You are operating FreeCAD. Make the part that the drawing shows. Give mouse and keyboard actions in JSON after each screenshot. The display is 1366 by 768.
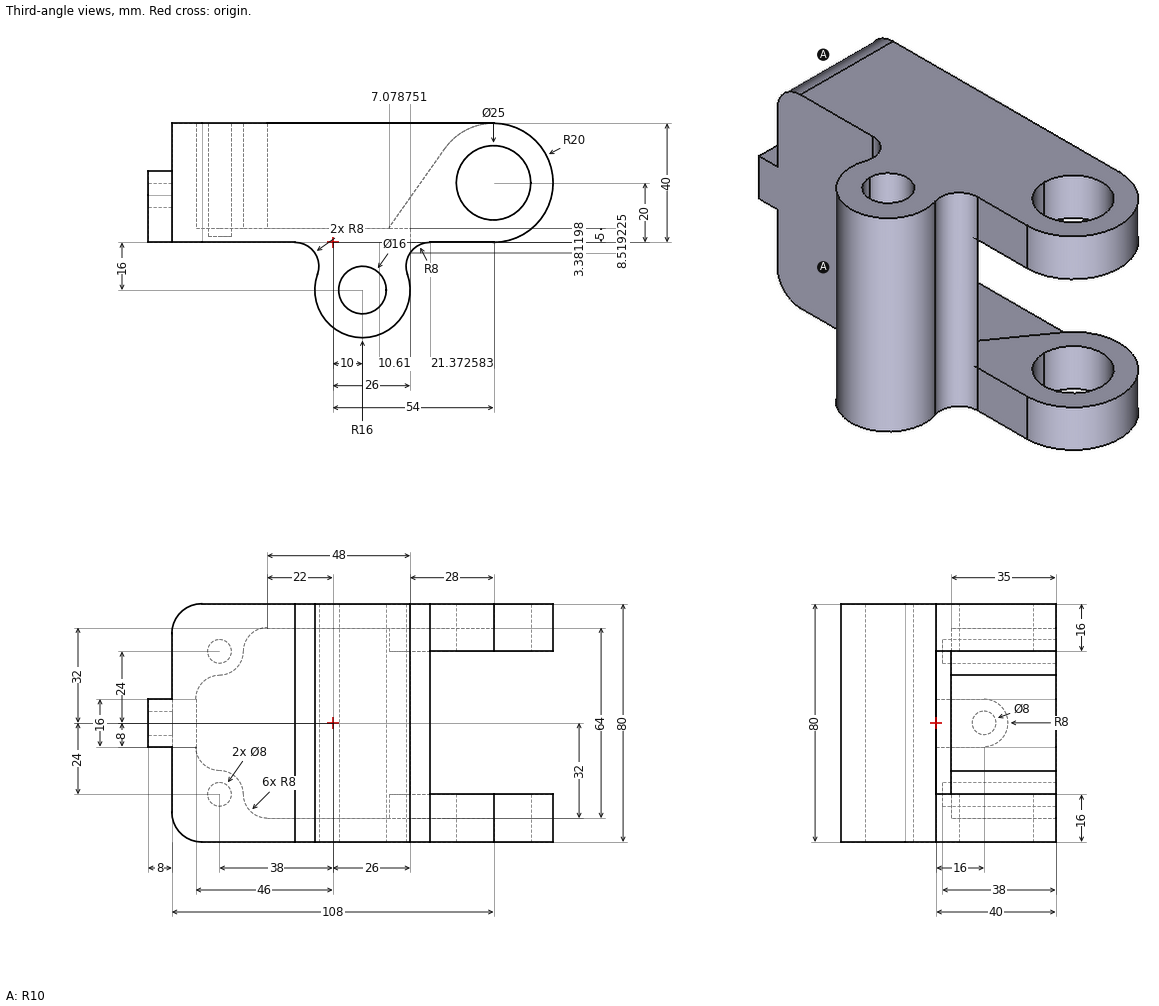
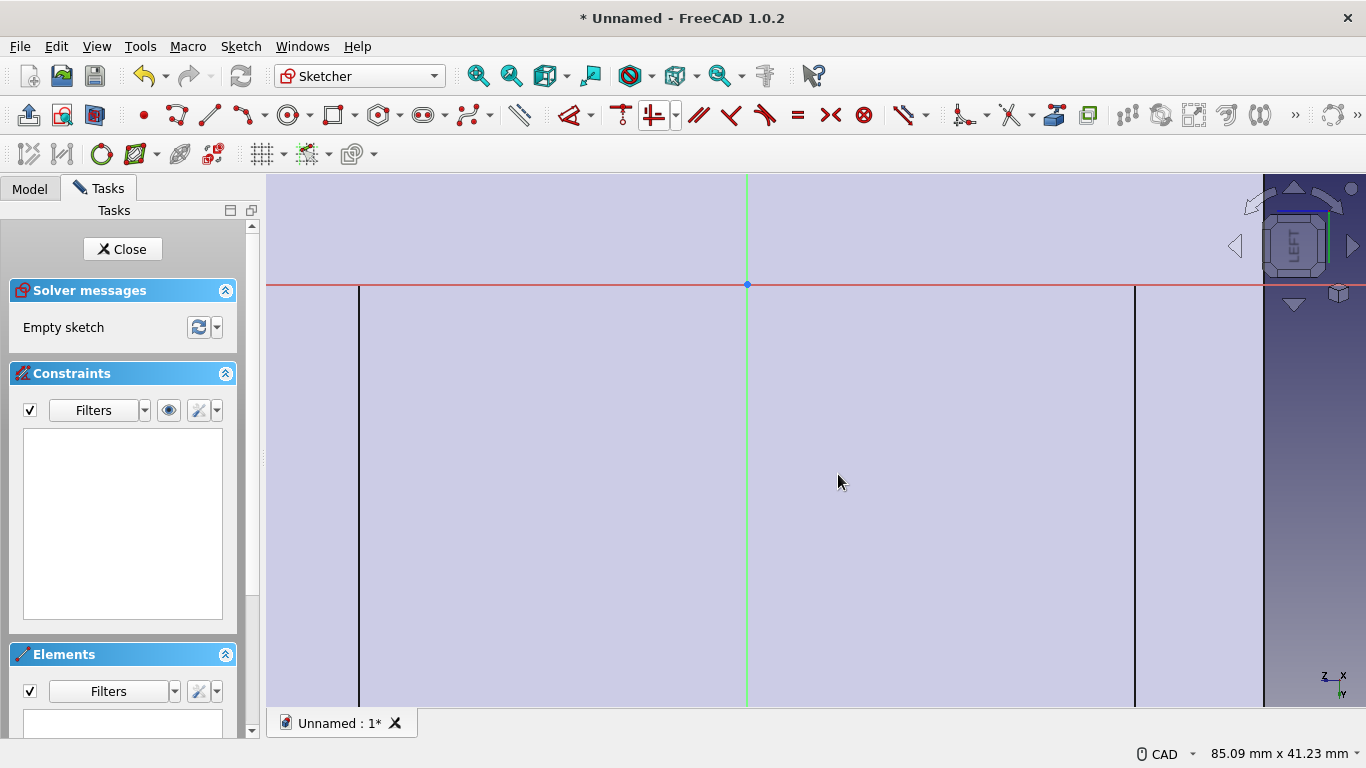
{"action": "key", "text": "g m"}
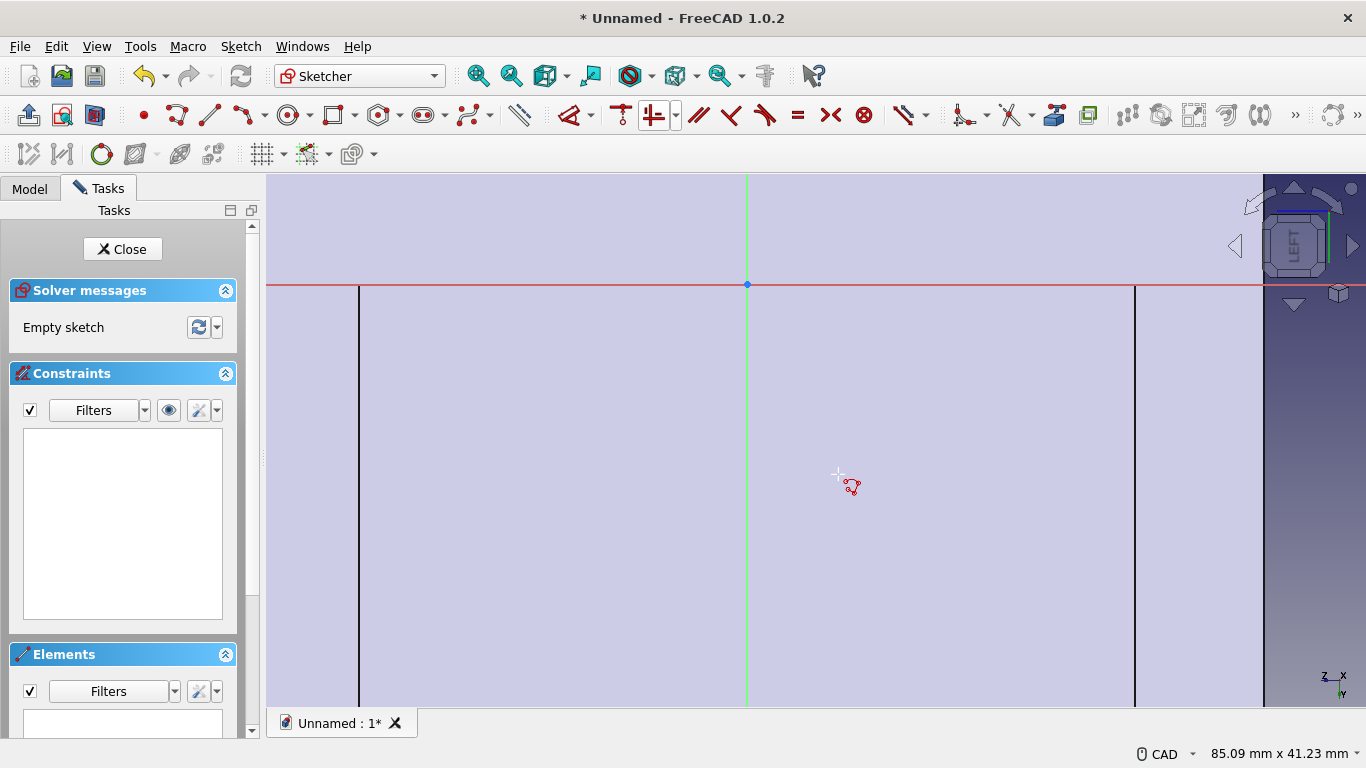
{"action": "left_click", "coordinate": [851, 492]}
{"action": "left_click", "coordinate": [851, 285]}
{"action": "left_click", "coordinate": [644, 294]}
{"action": "left_click", "coordinate": [644, 492]}
{"action": "right_click", "coordinate": [644, 492]}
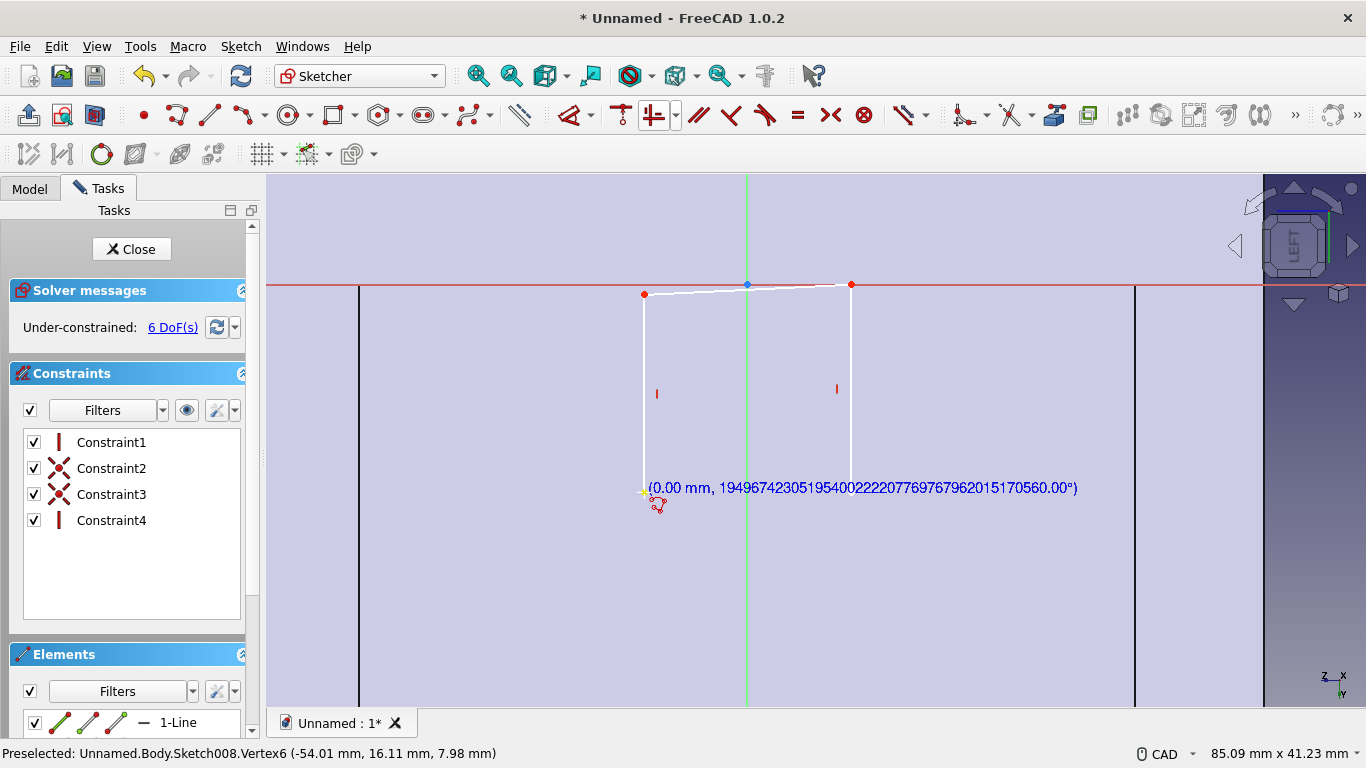
{"action": "left_click", "coordinate": [242, 116]}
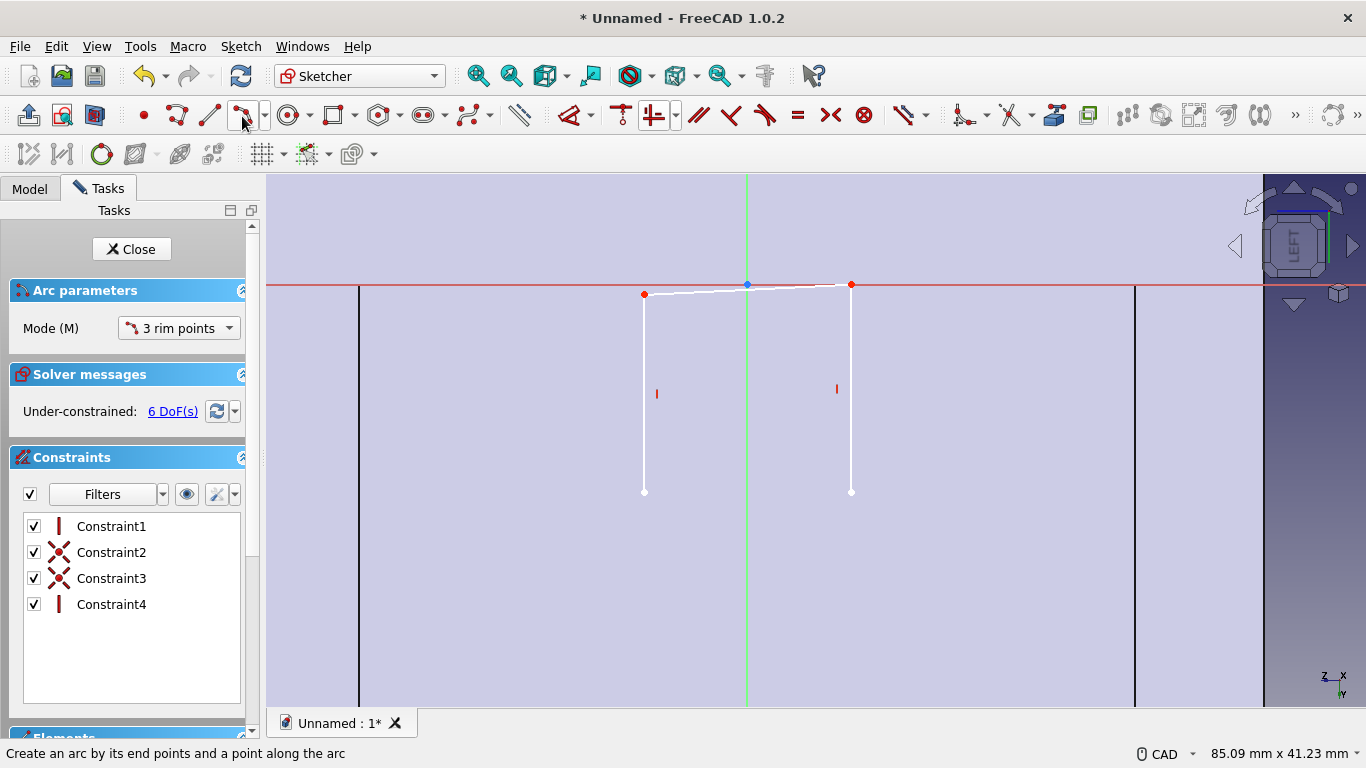
{"action": "left_click", "coordinate": [644, 493]}
{"action": "left_click", "coordinate": [851, 493]}
{"action": "left_click", "coordinate": [715, 590]}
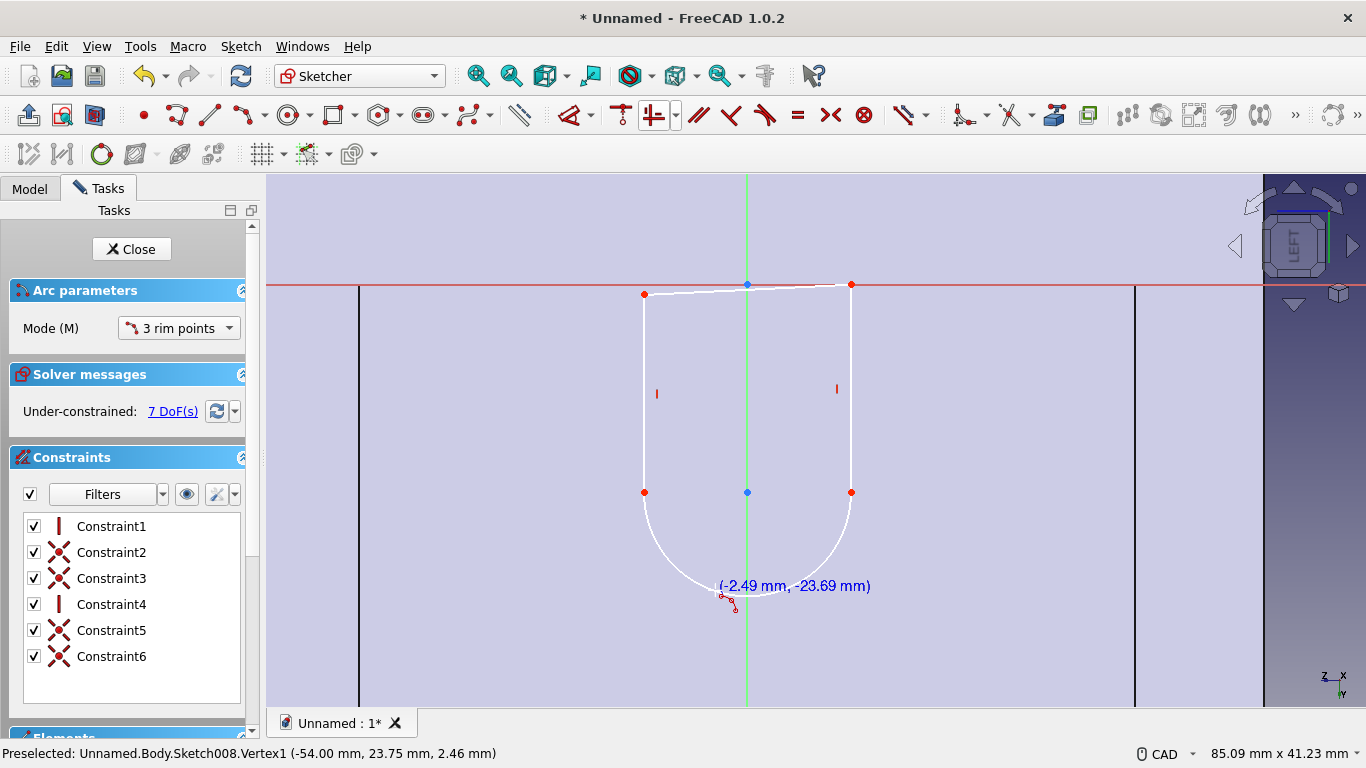
{"action": "key", "text": "g c"}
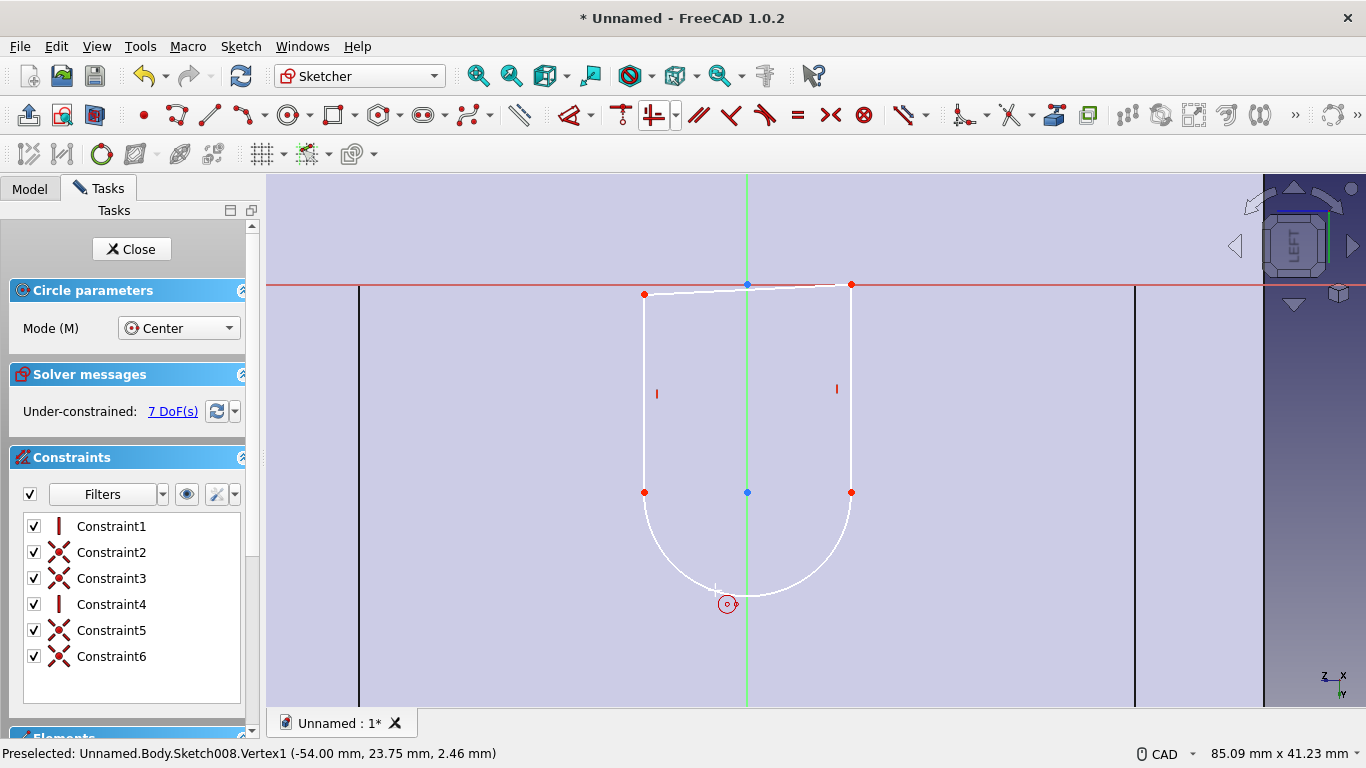
{"action": "left_click", "coordinate": [747, 492]}
{"action": "mouse_move", "coordinate": [784, 455]}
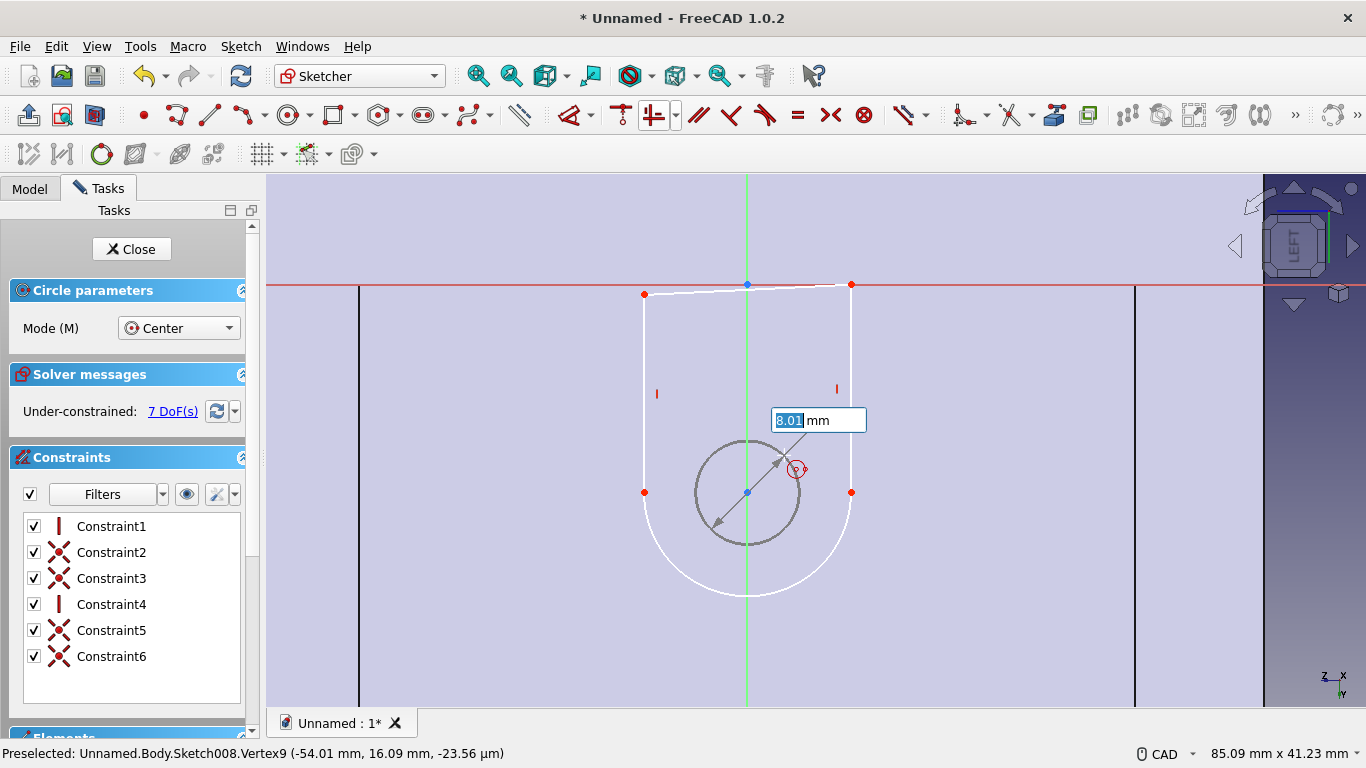
{"action": "type", "text": "8"}
{"action": "key", "text": "Return"}
{"action": "key", "text": "Escape"}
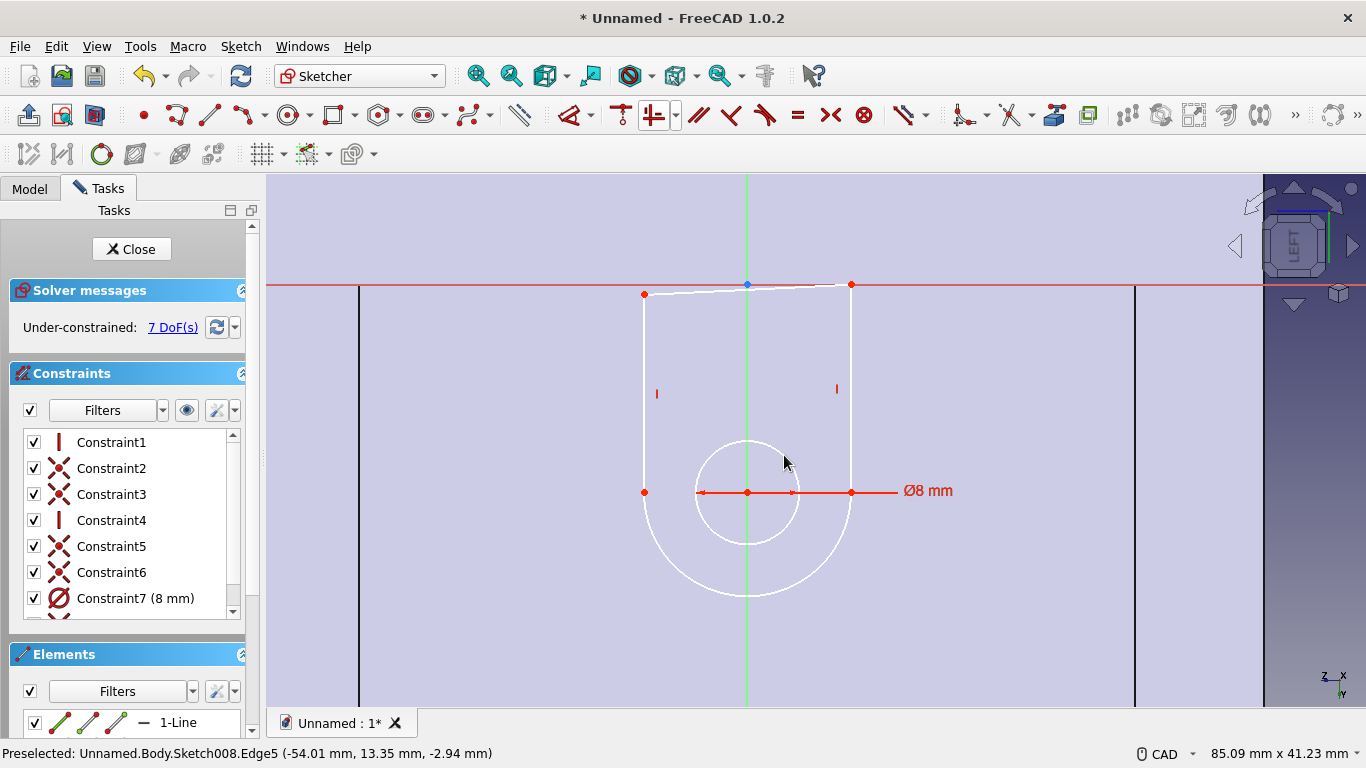
{"action": "left_click", "coordinate": [851, 431]}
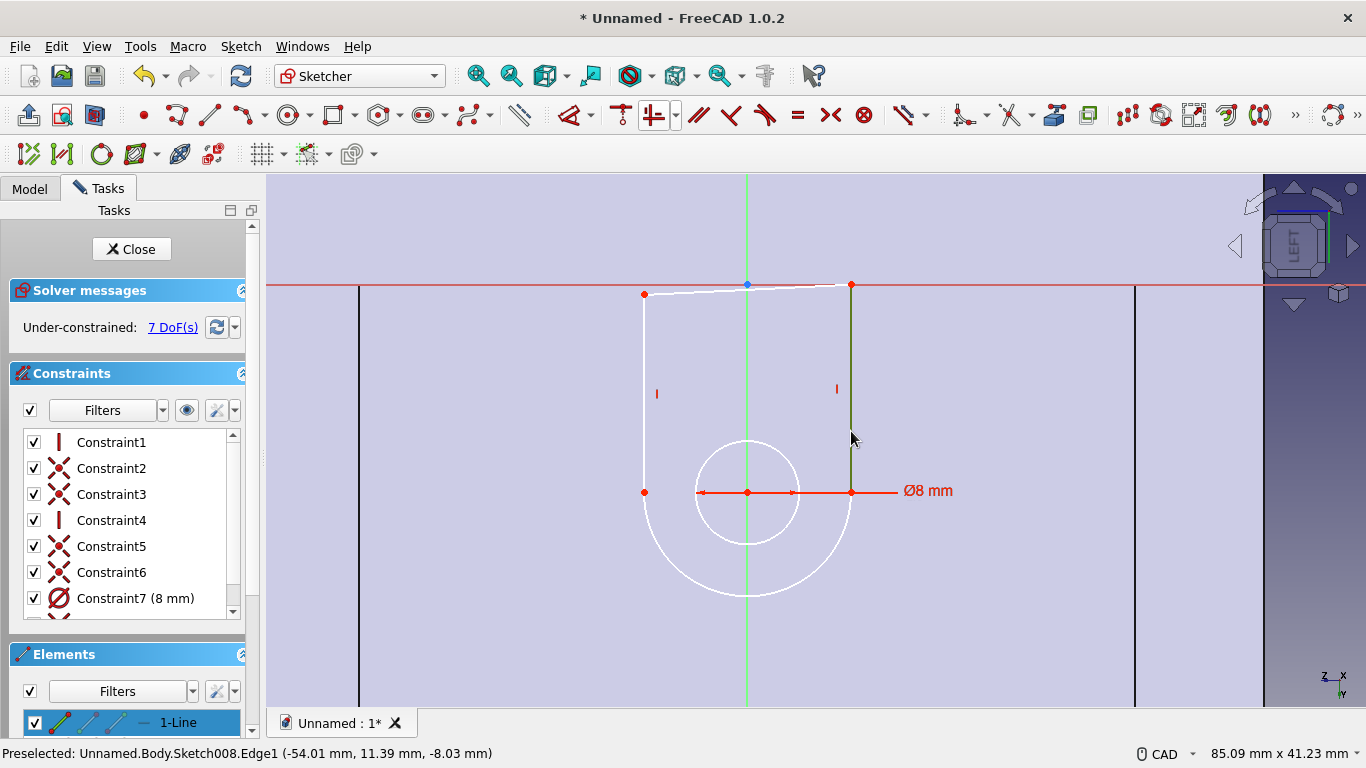
{"action": "left_click", "coordinate": [687, 577]}